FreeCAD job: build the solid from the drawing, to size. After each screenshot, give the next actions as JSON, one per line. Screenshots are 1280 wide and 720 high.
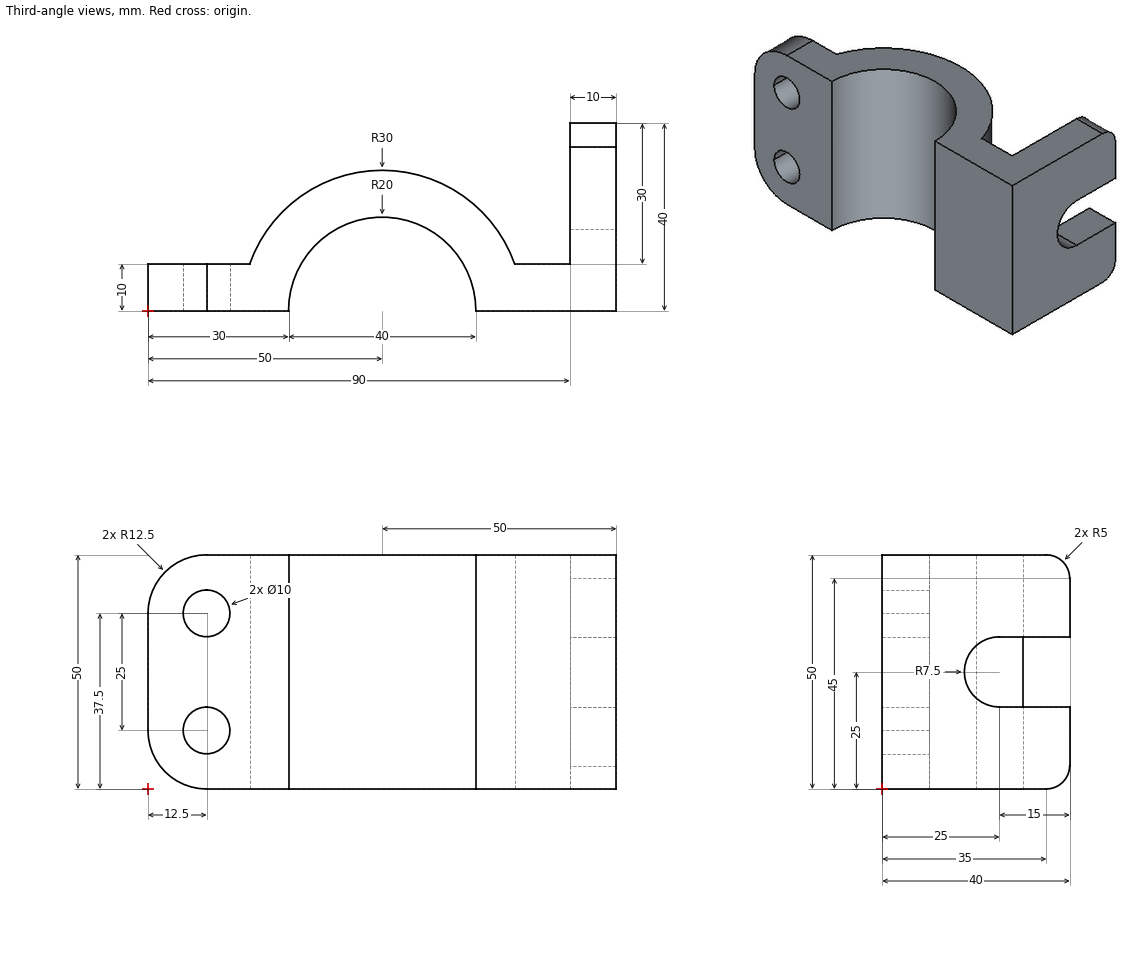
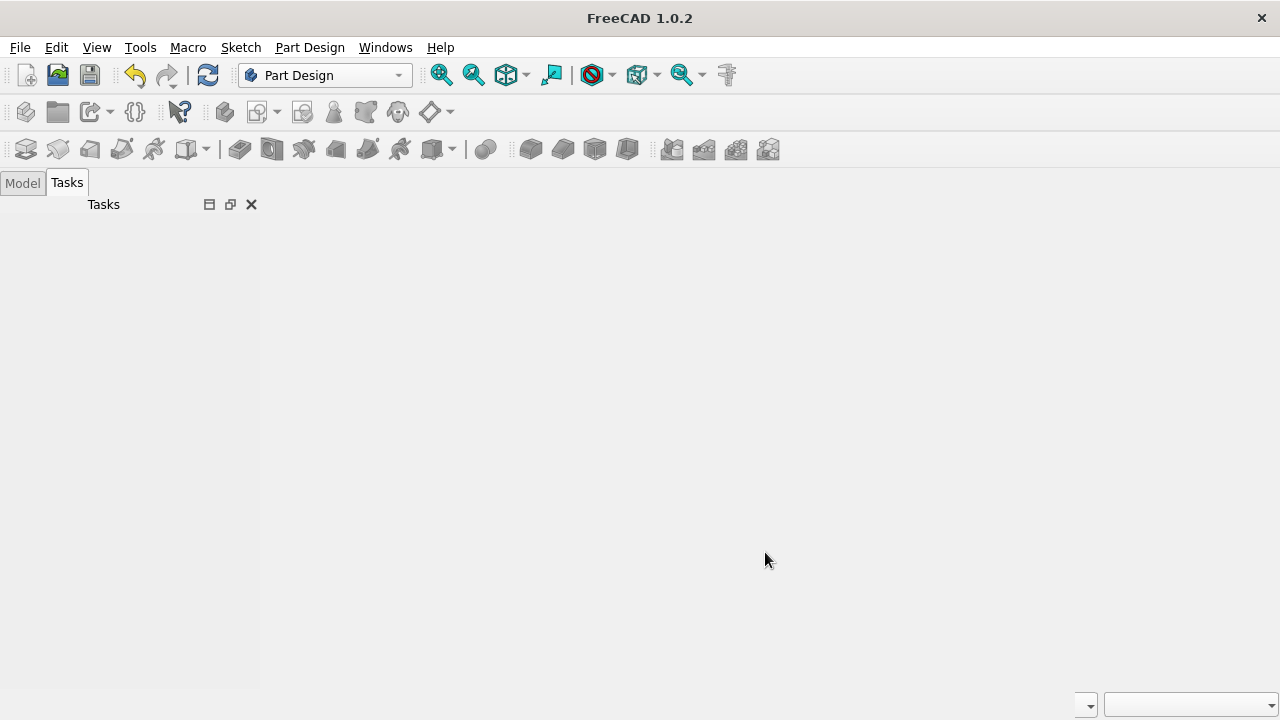
{"action": "left_click", "coordinate": [26, 76]}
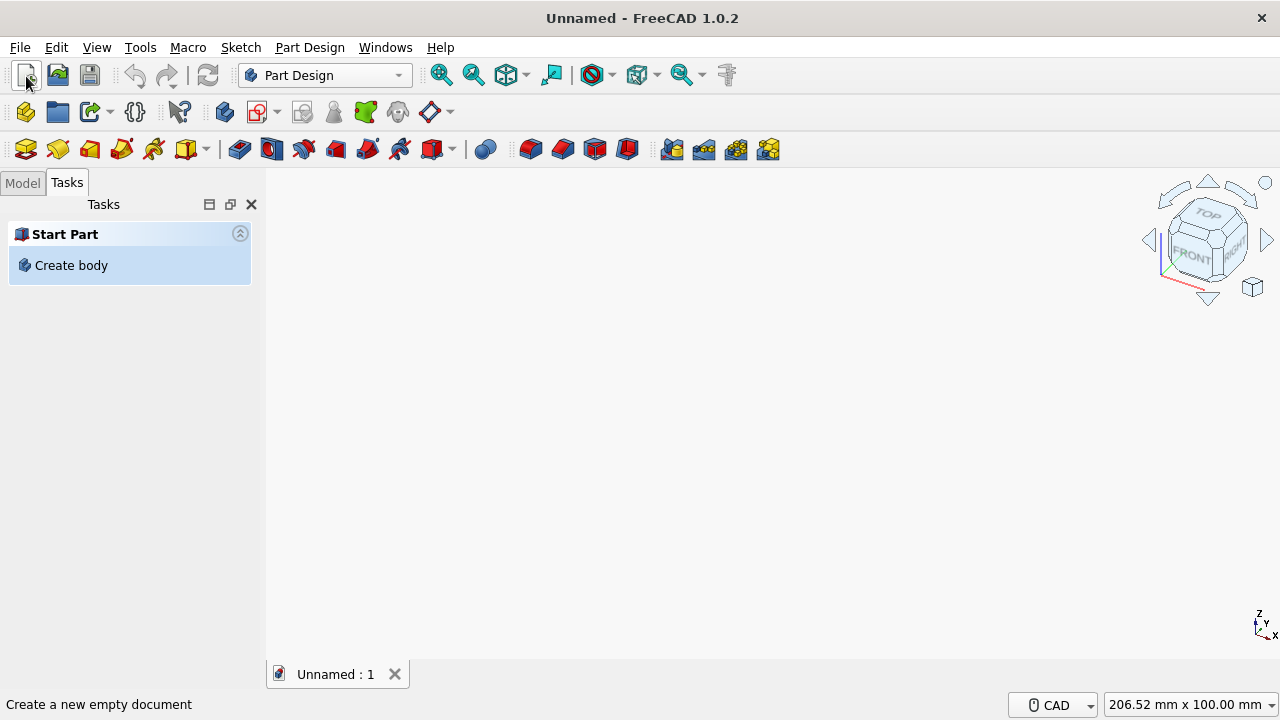
{"action": "left_click", "coordinate": [258, 112]}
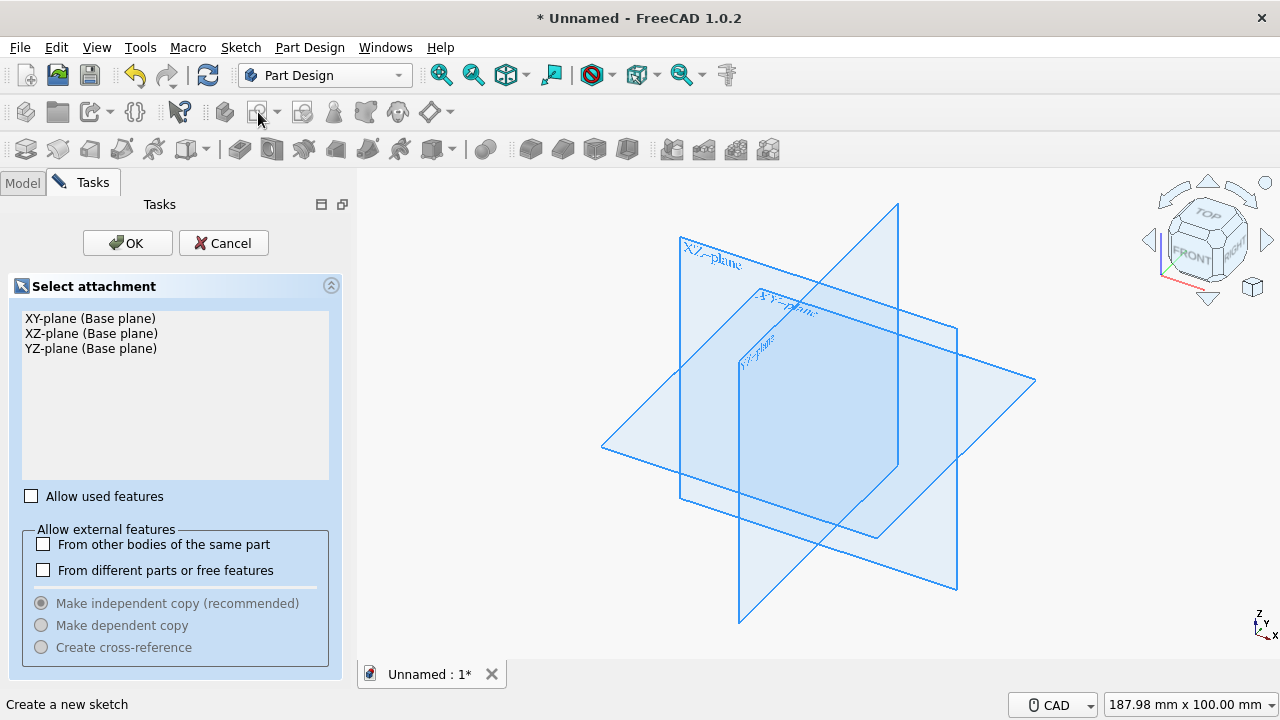
{"action": "left_click", "coordinate": [82, 318]}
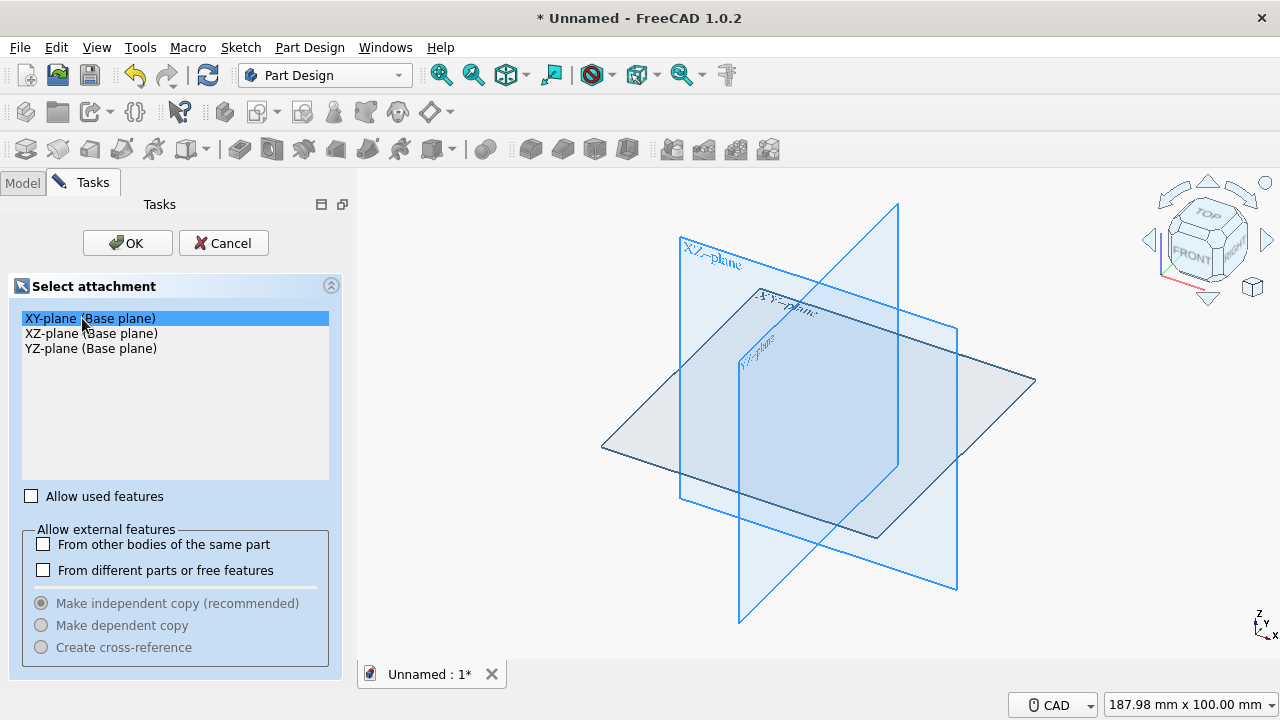
{"action": "left_click", "coordinate": [128, 243]}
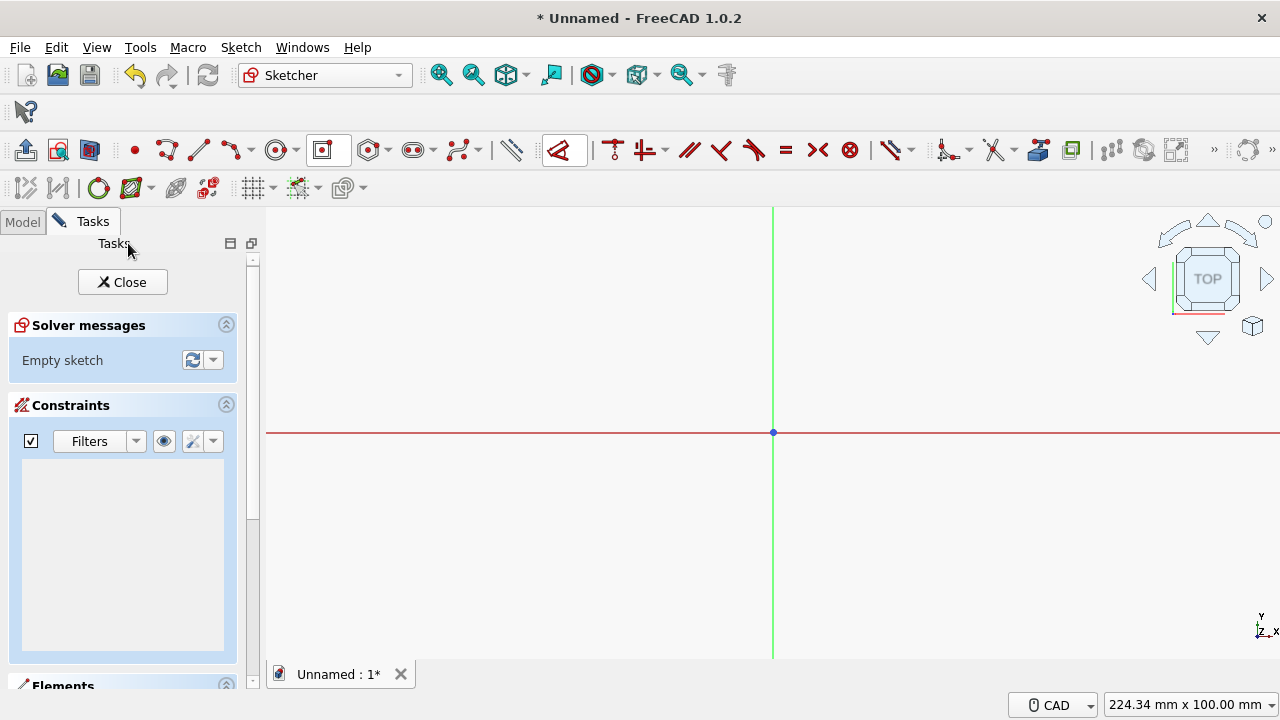
{"action": "scroll", "coordinate": [294, 631], "scroll_direction": "down", "scroll_amount": 1}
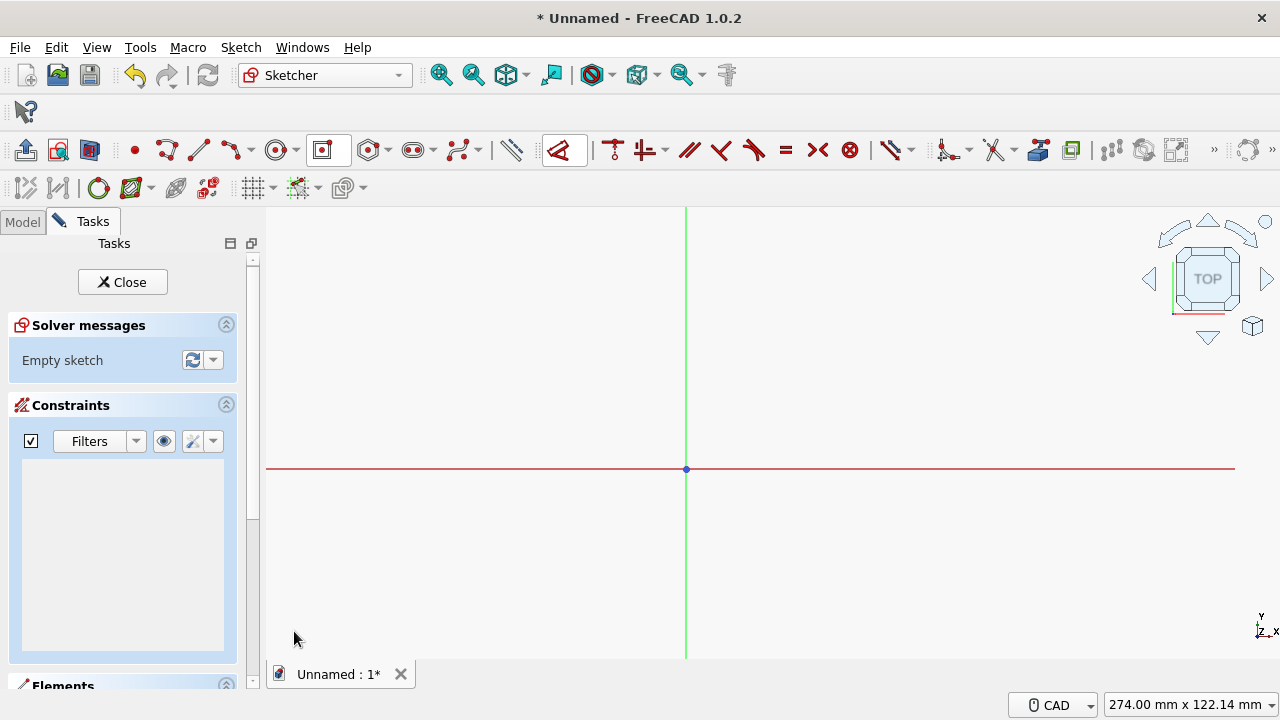
{"action": "scroll", "coordinate": [1115, 318], "scroll_direction": "up", "scroll_amount": 2}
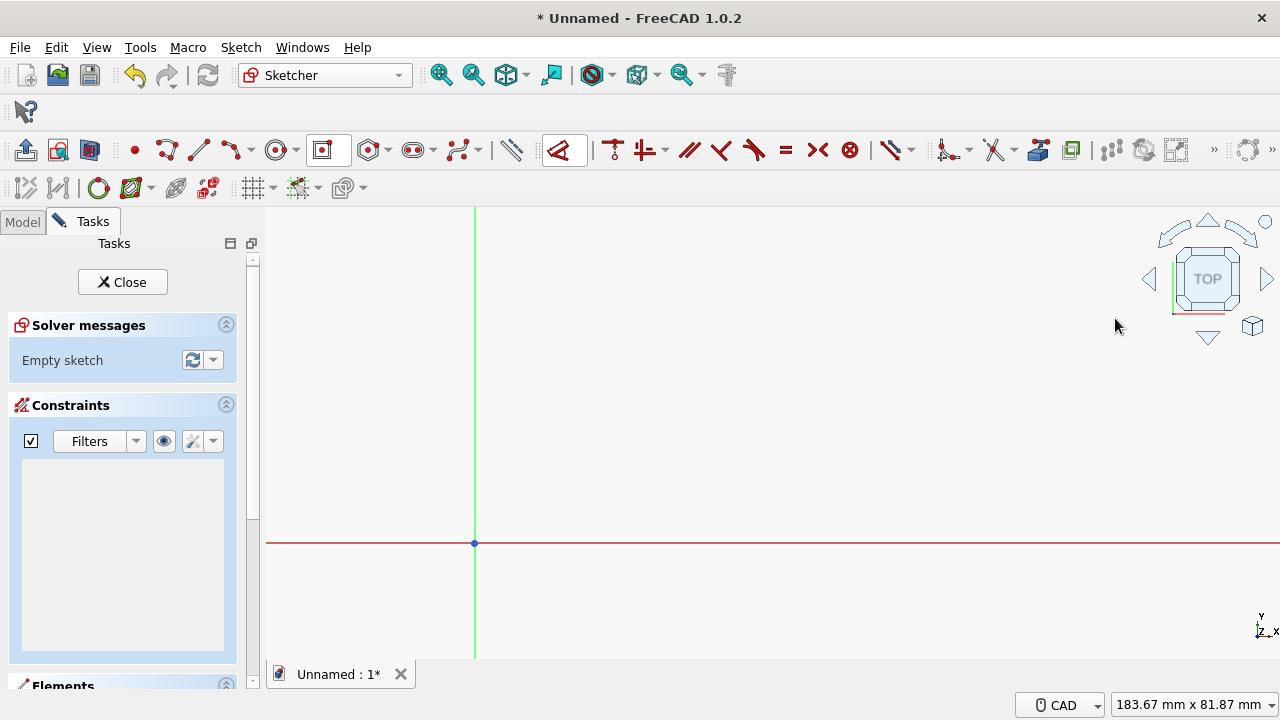
{"action": "left_click", "coordinate": [168, 150]}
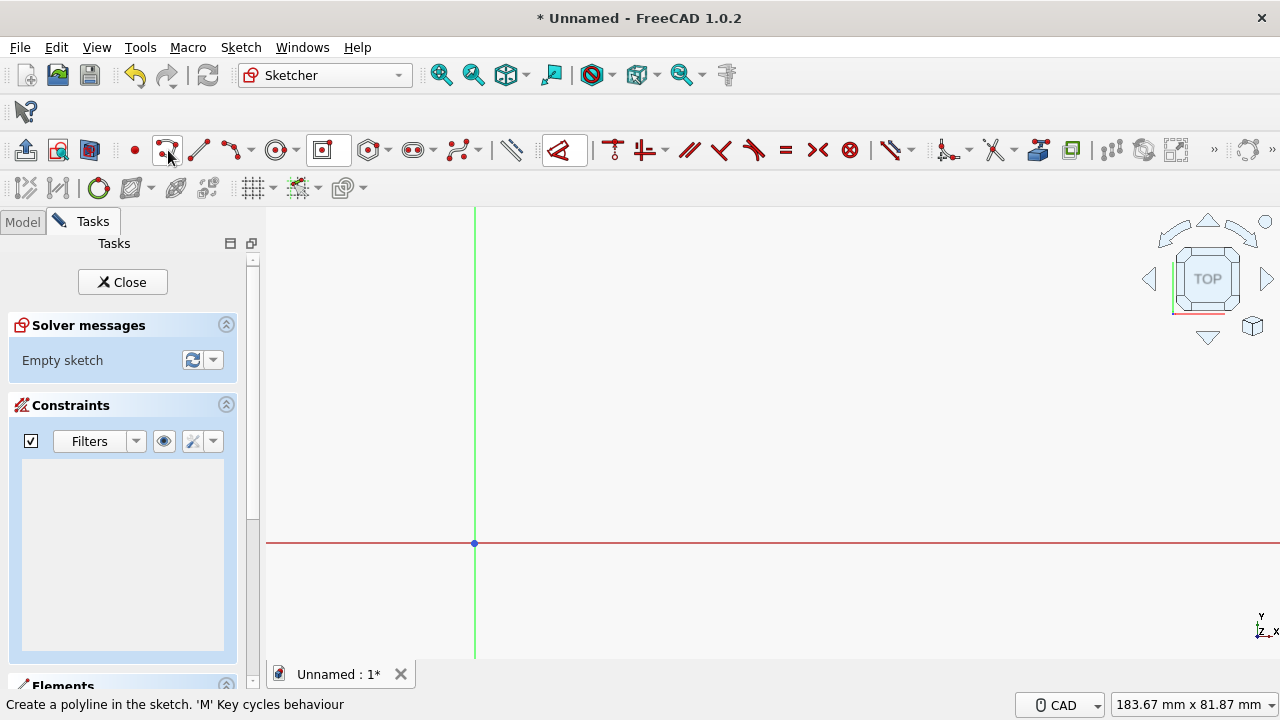
{"action": "left_click", "coordinate": [475, 543]}
{"action": "left_click", "coordinate": [1027, 534]}
{"action": "left_click", "coordinate": [1027, 322]}
{"action": "left_click", "coordinate": [972, 322]}
{"action": "left_click", "coordinate": [972, 488]}
{"action": "left_click", "coordinate": [484, 488]}
{"action": "left_click", "coordinate": [475, 543]}
{"action": "key", "text": "Escape"}
{"action": "key", "text": "Escape"}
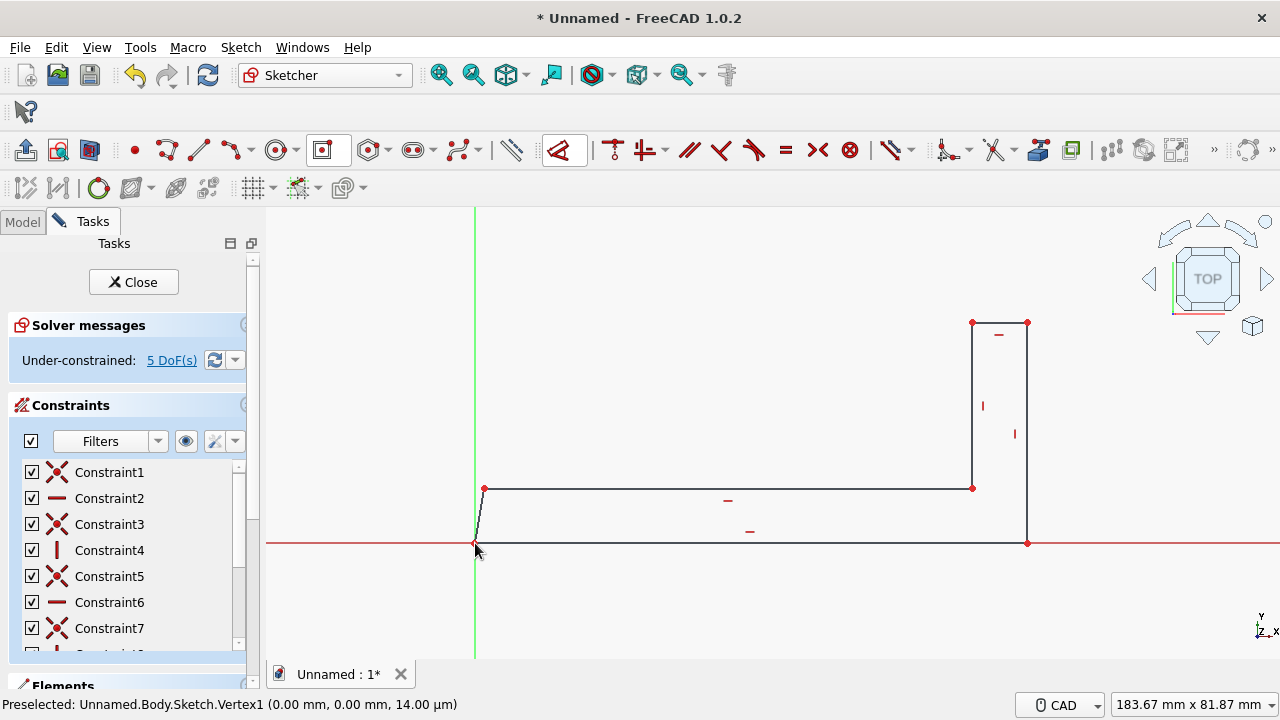
{"action": "left_click", "coordinate": [478, 527]}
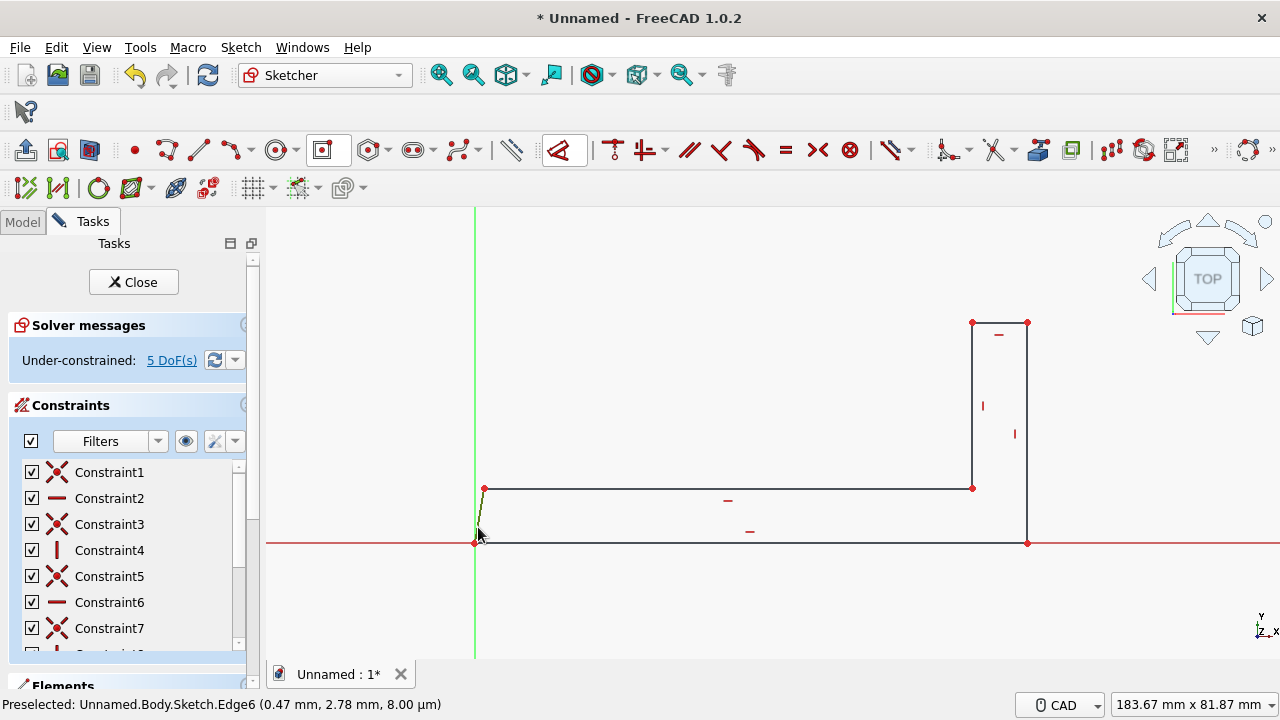
{"action": "left_click", "coordinate": [668, 150]}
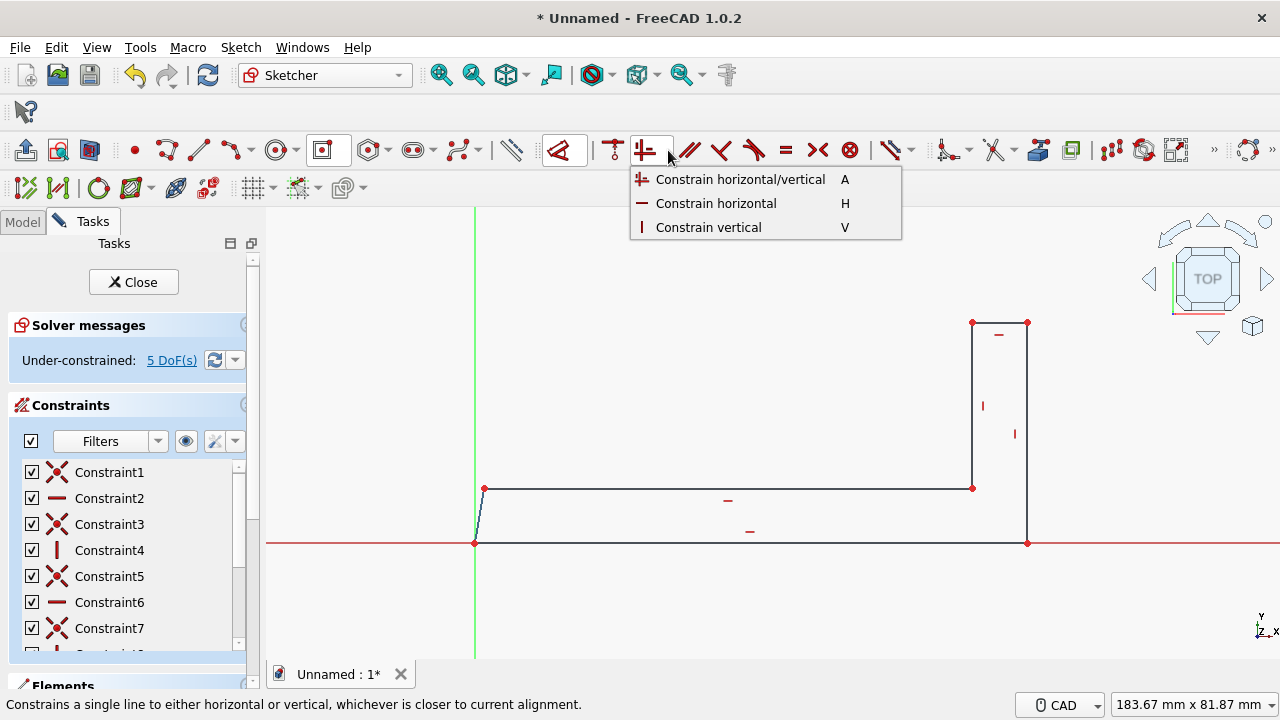
{"action": "left_click", "coordinate": [766, 227]}